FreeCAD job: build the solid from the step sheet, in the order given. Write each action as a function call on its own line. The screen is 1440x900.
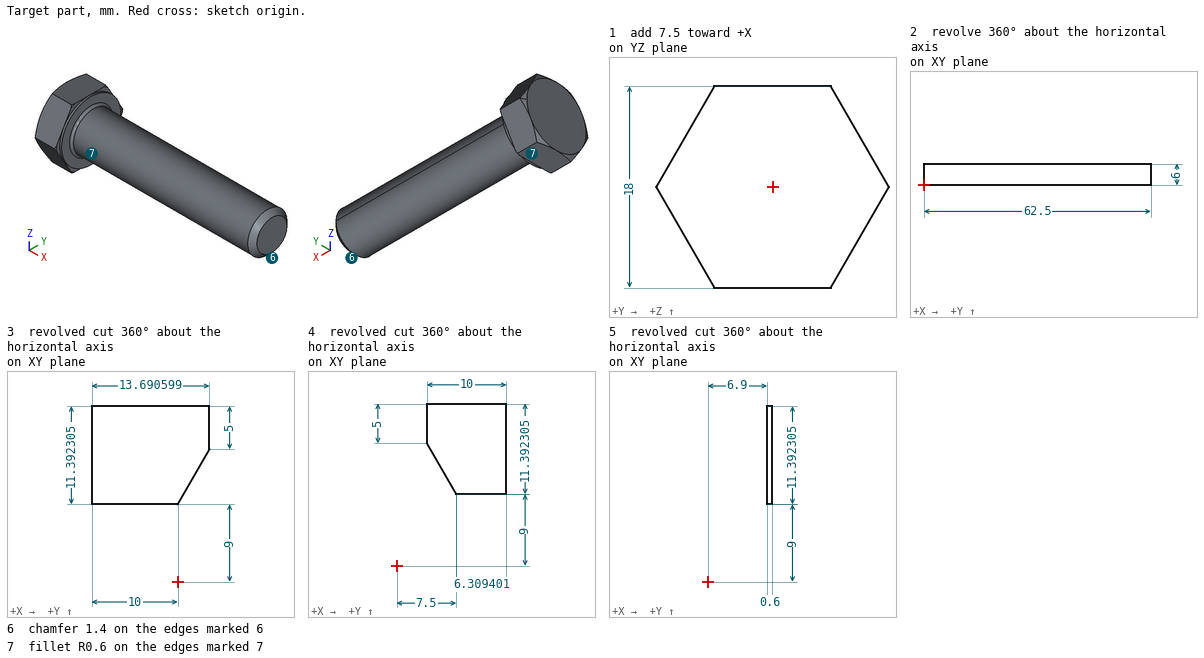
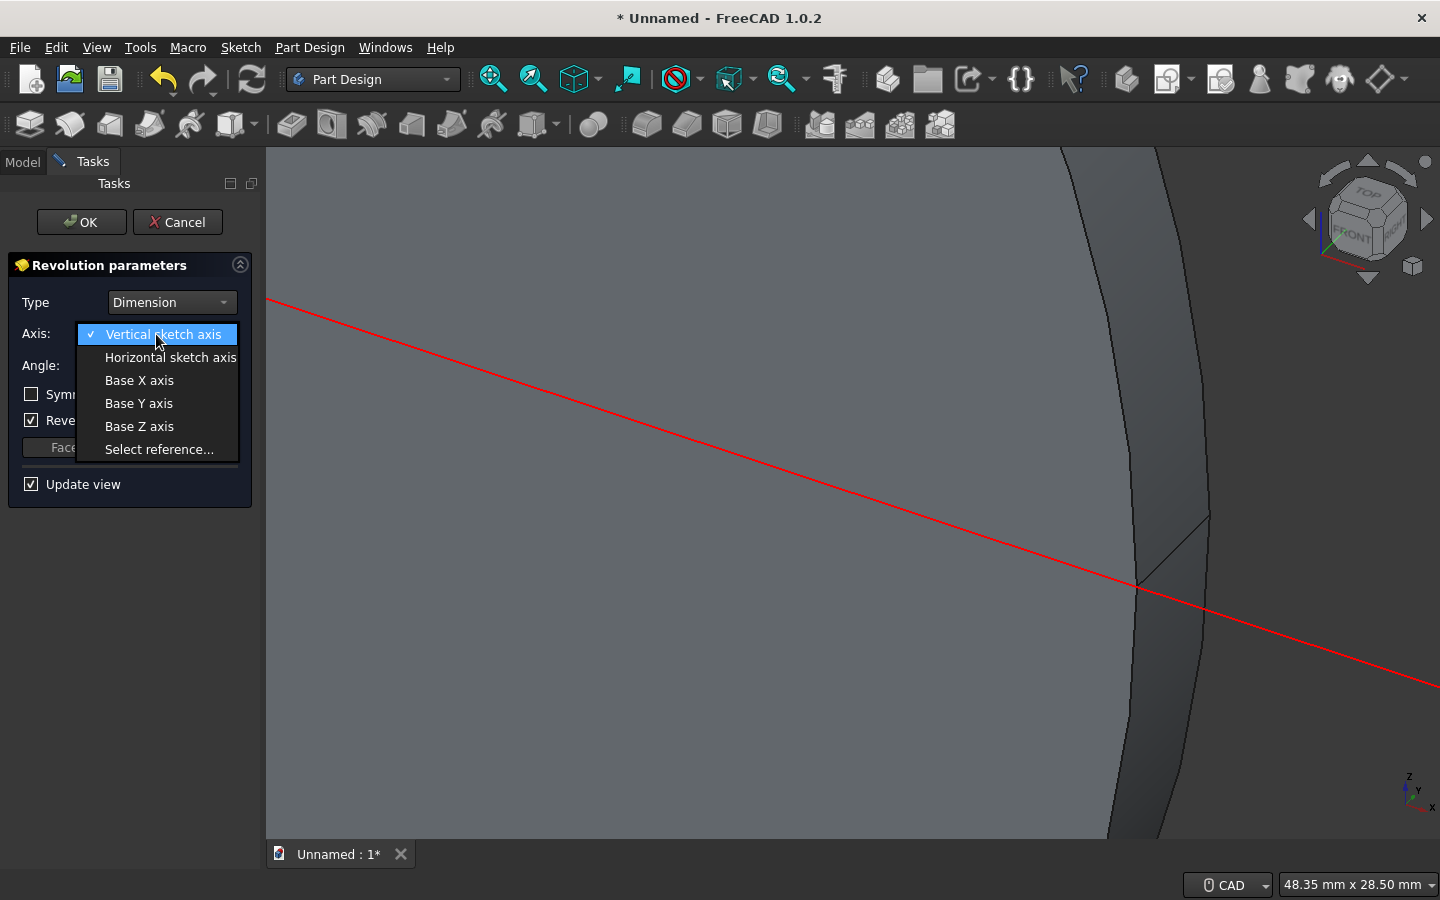
click(156, 358)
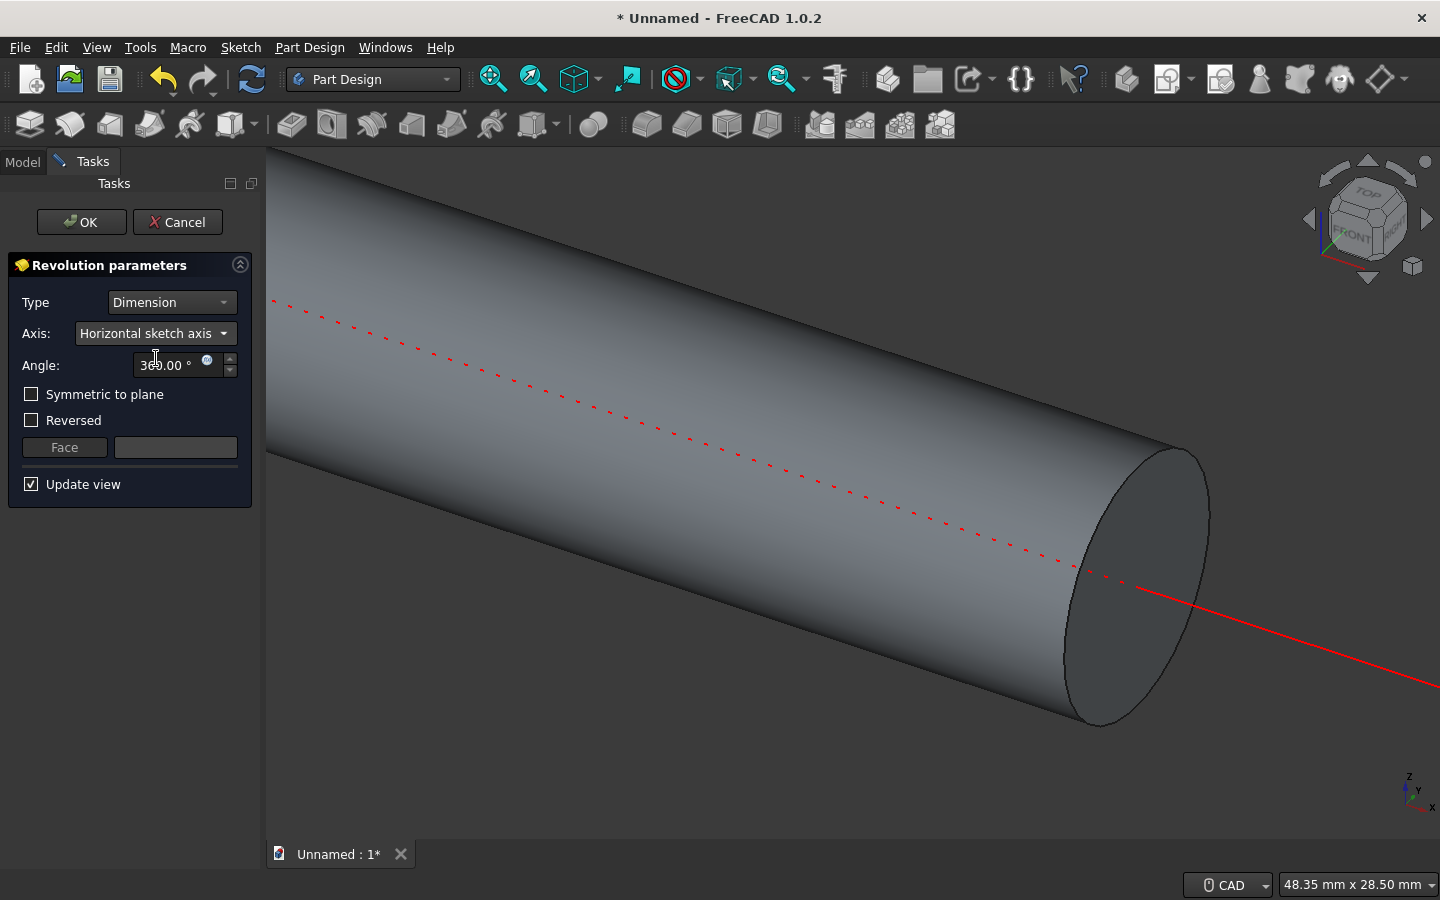
click(82, 222)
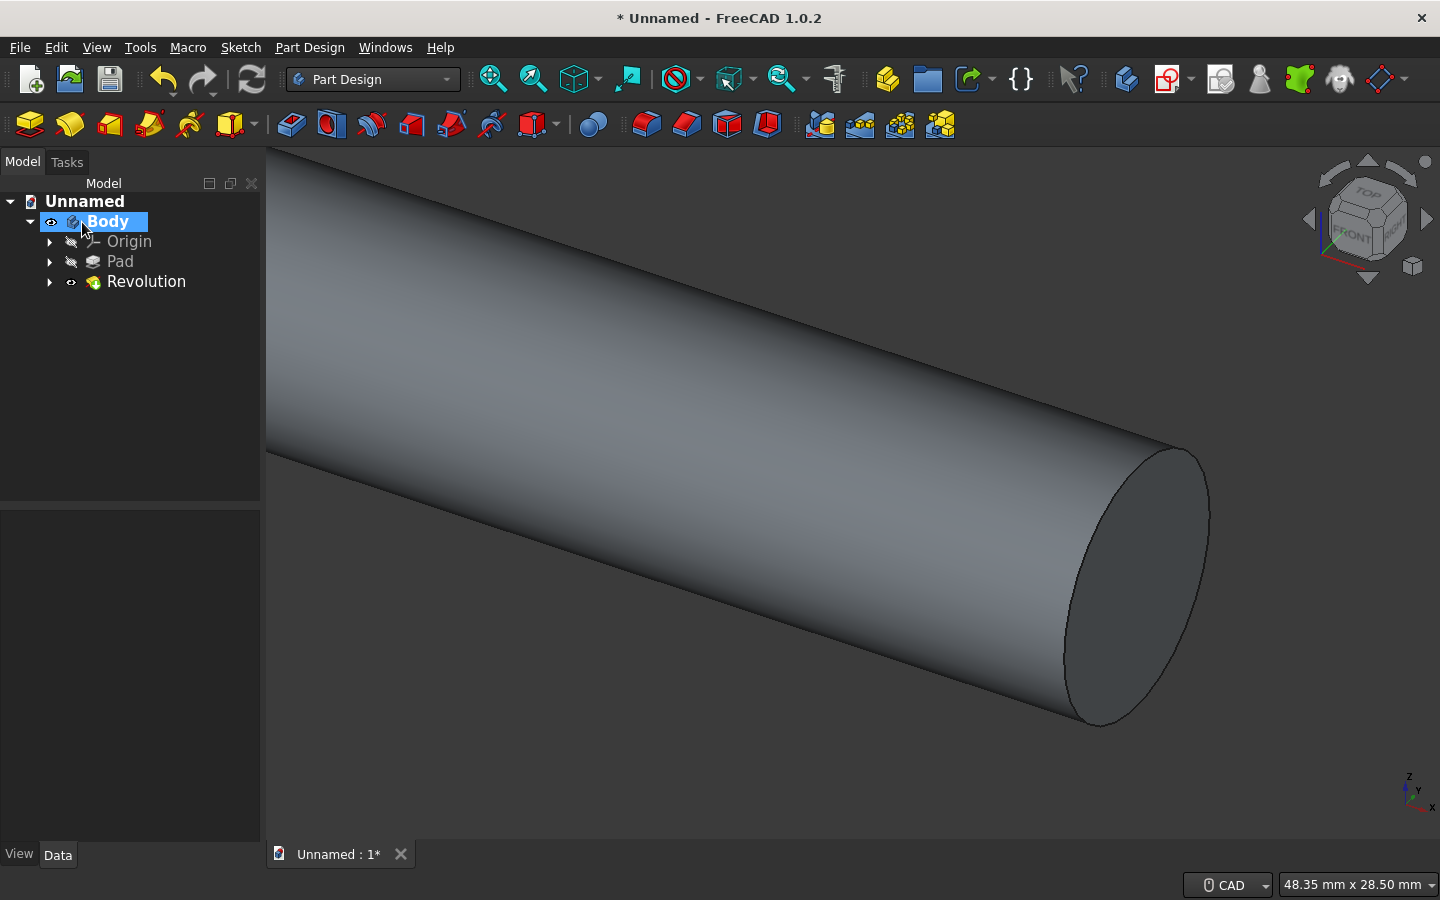
click(494, 80)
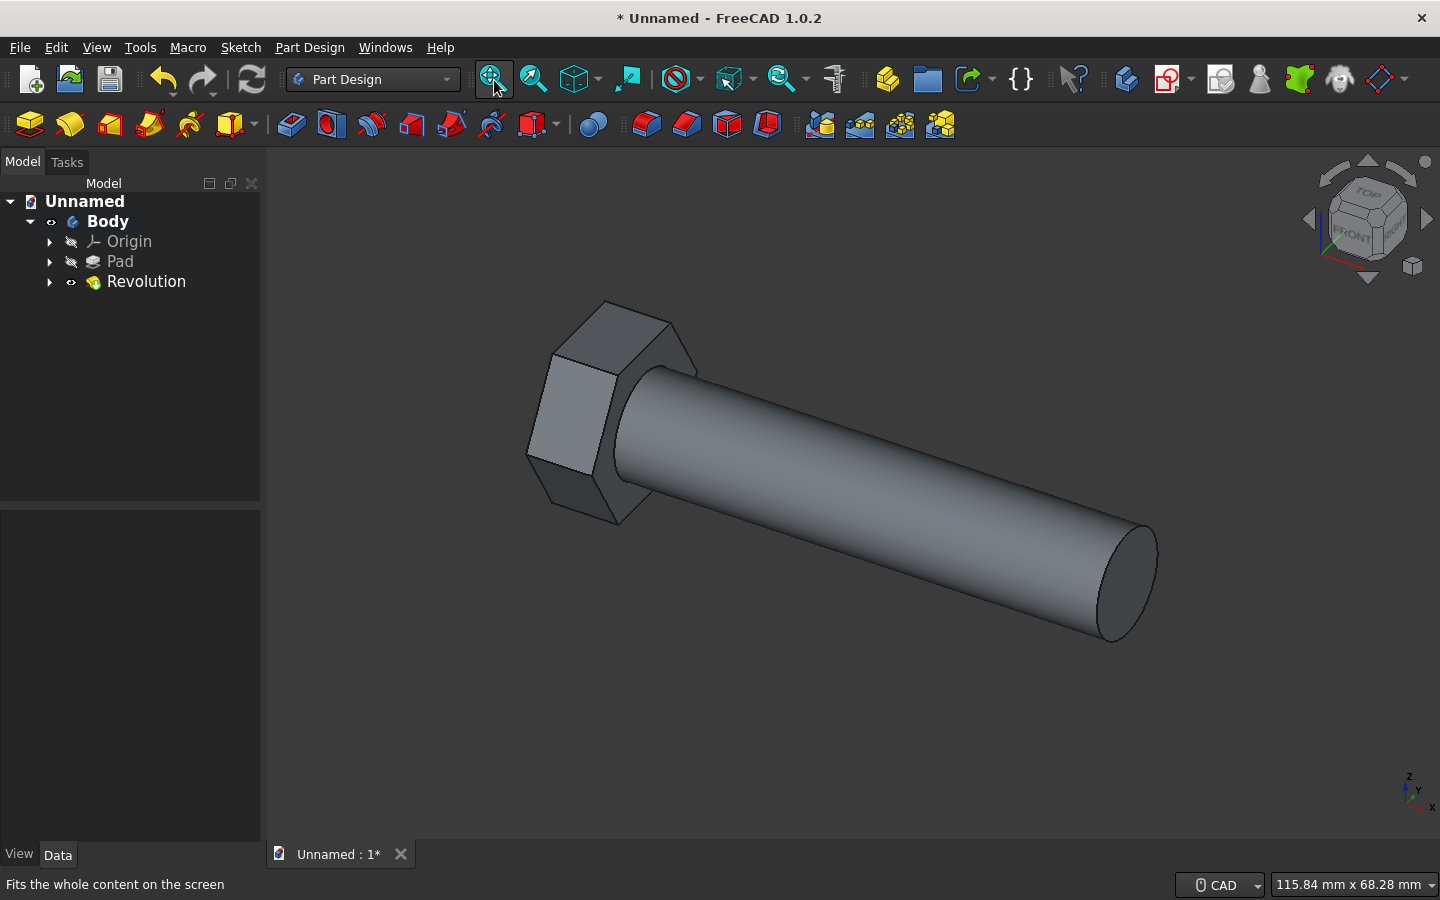
click(1168, 80)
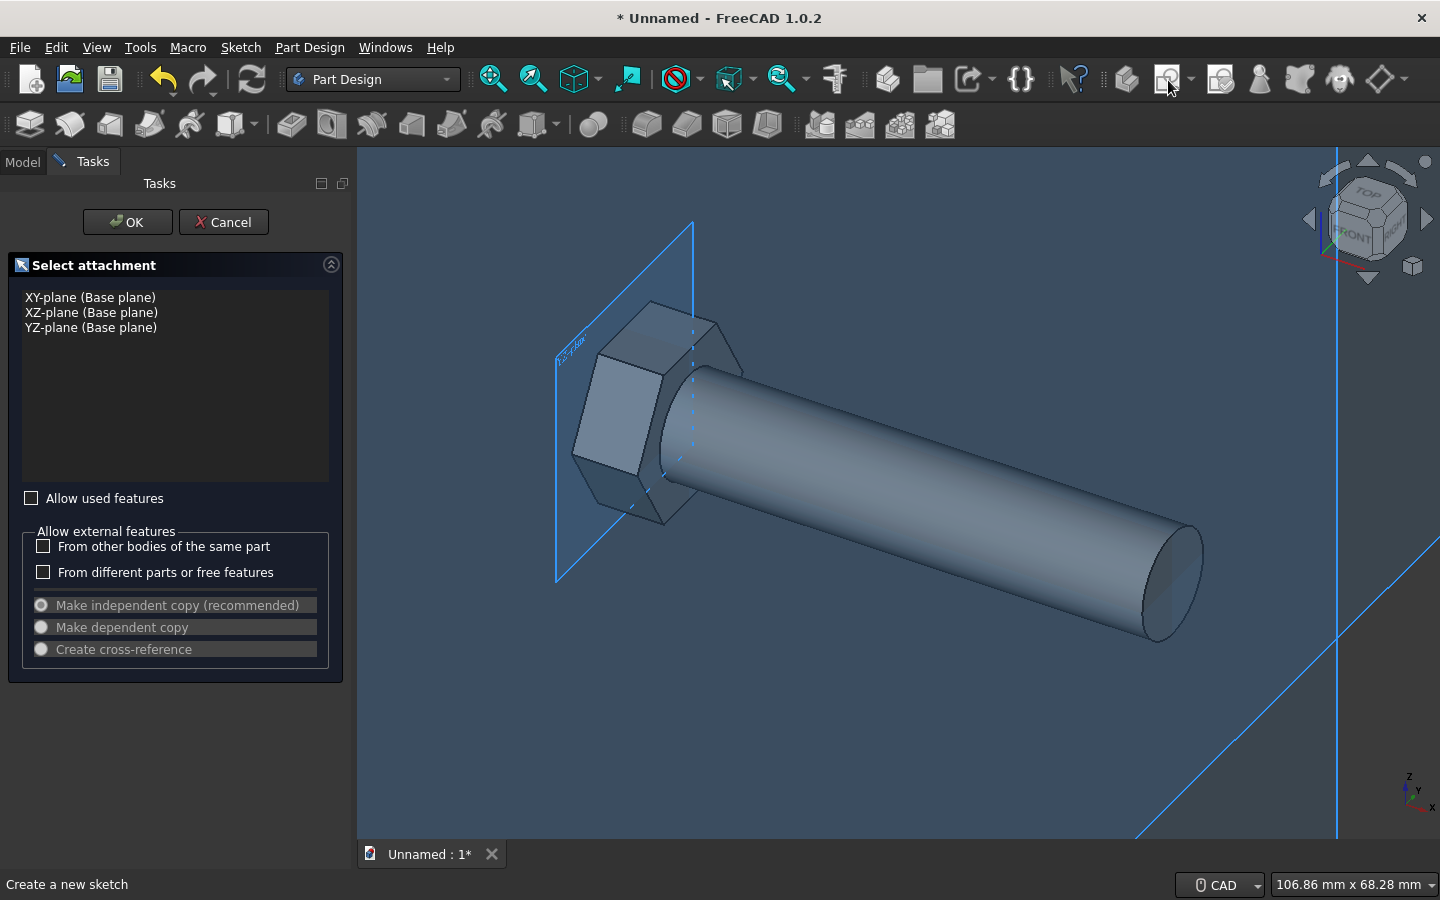
click(82, 298)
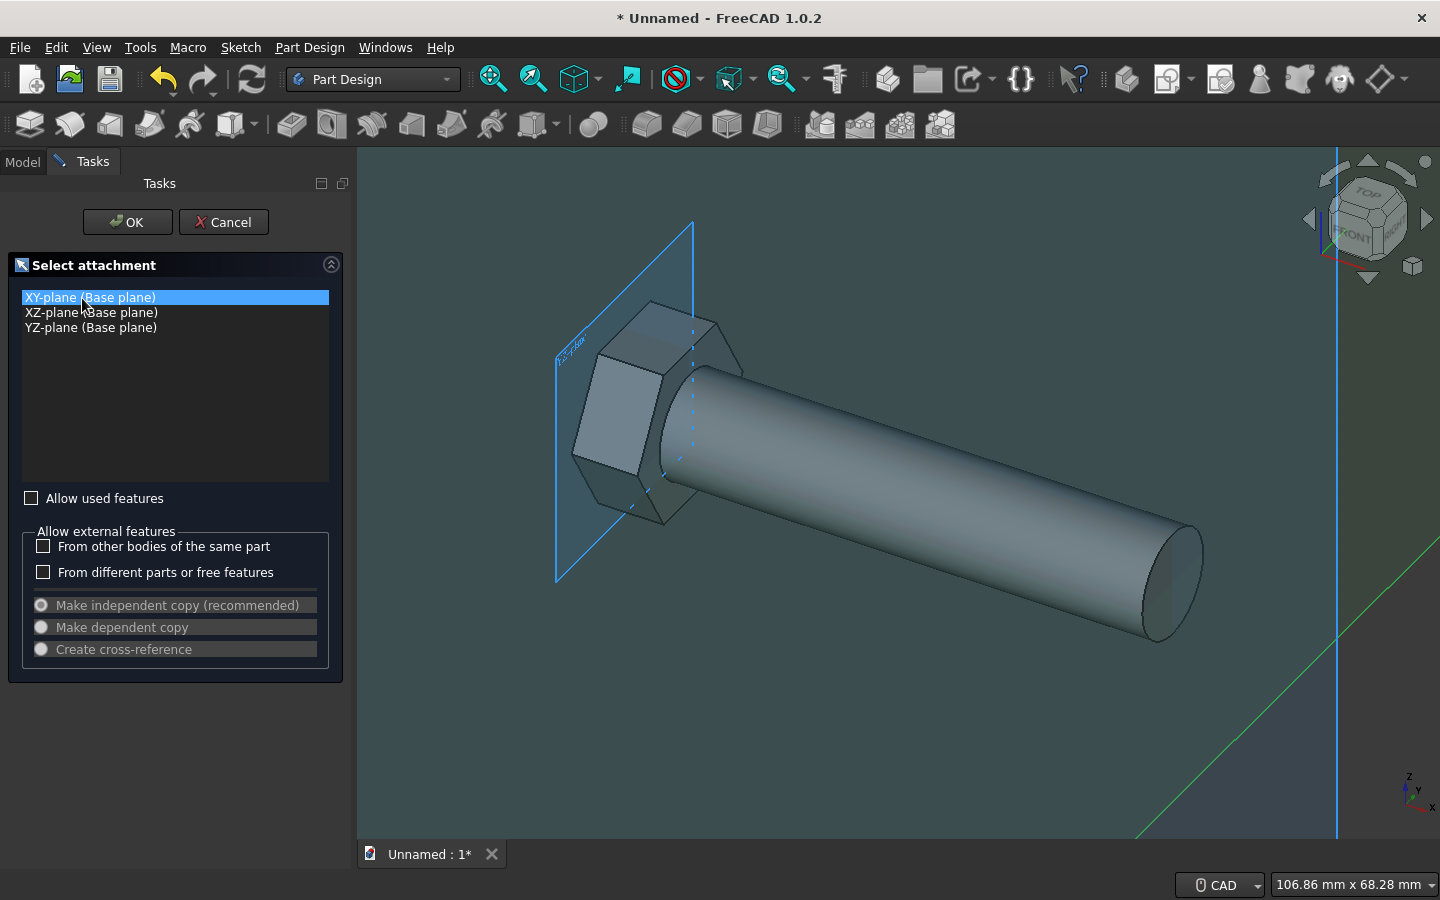
click(128, 222)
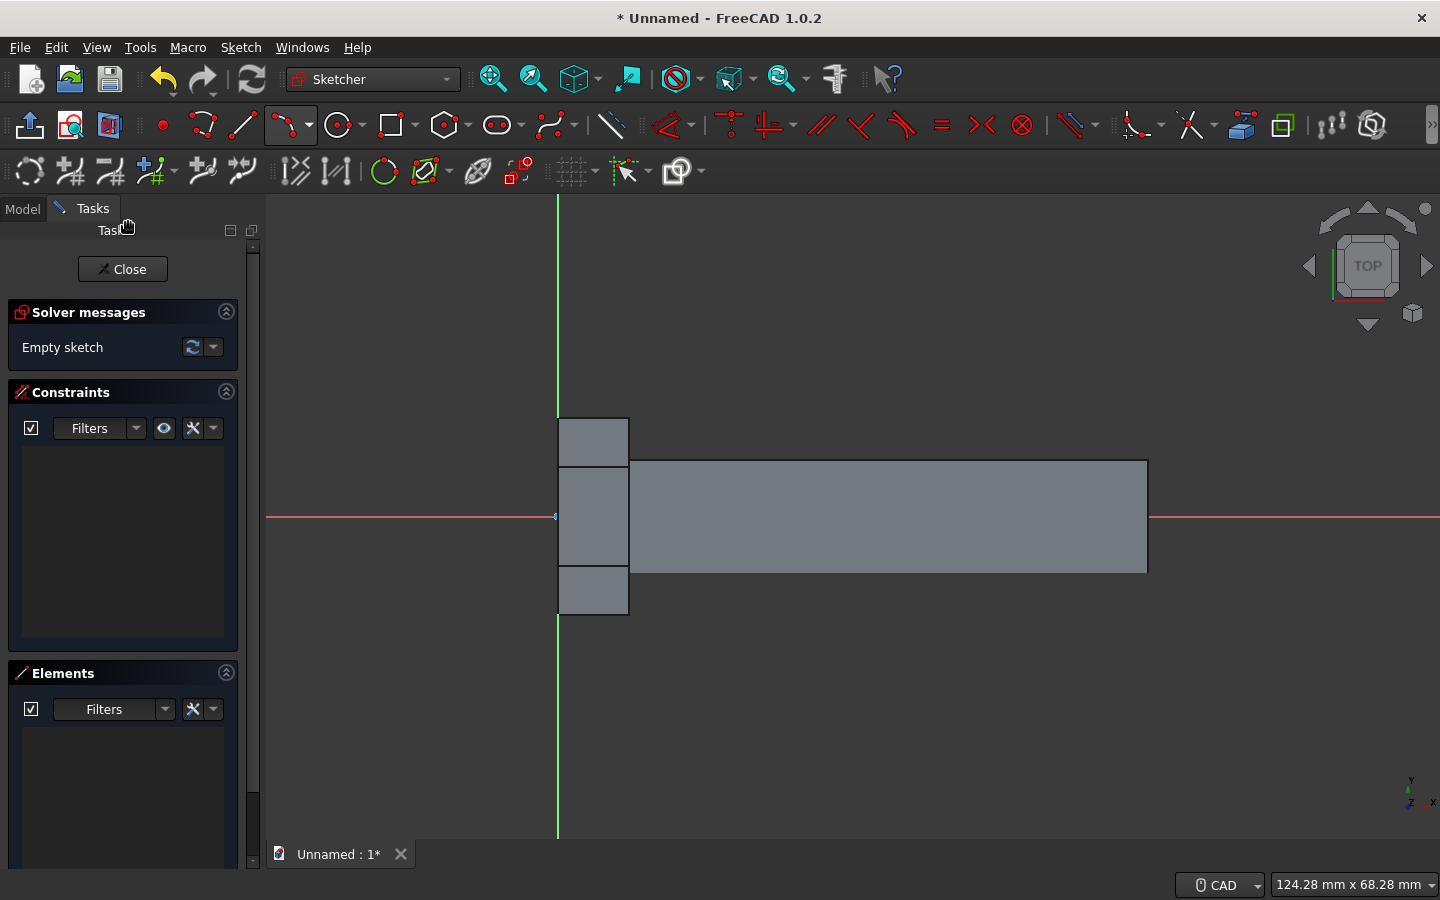
click(110, 126)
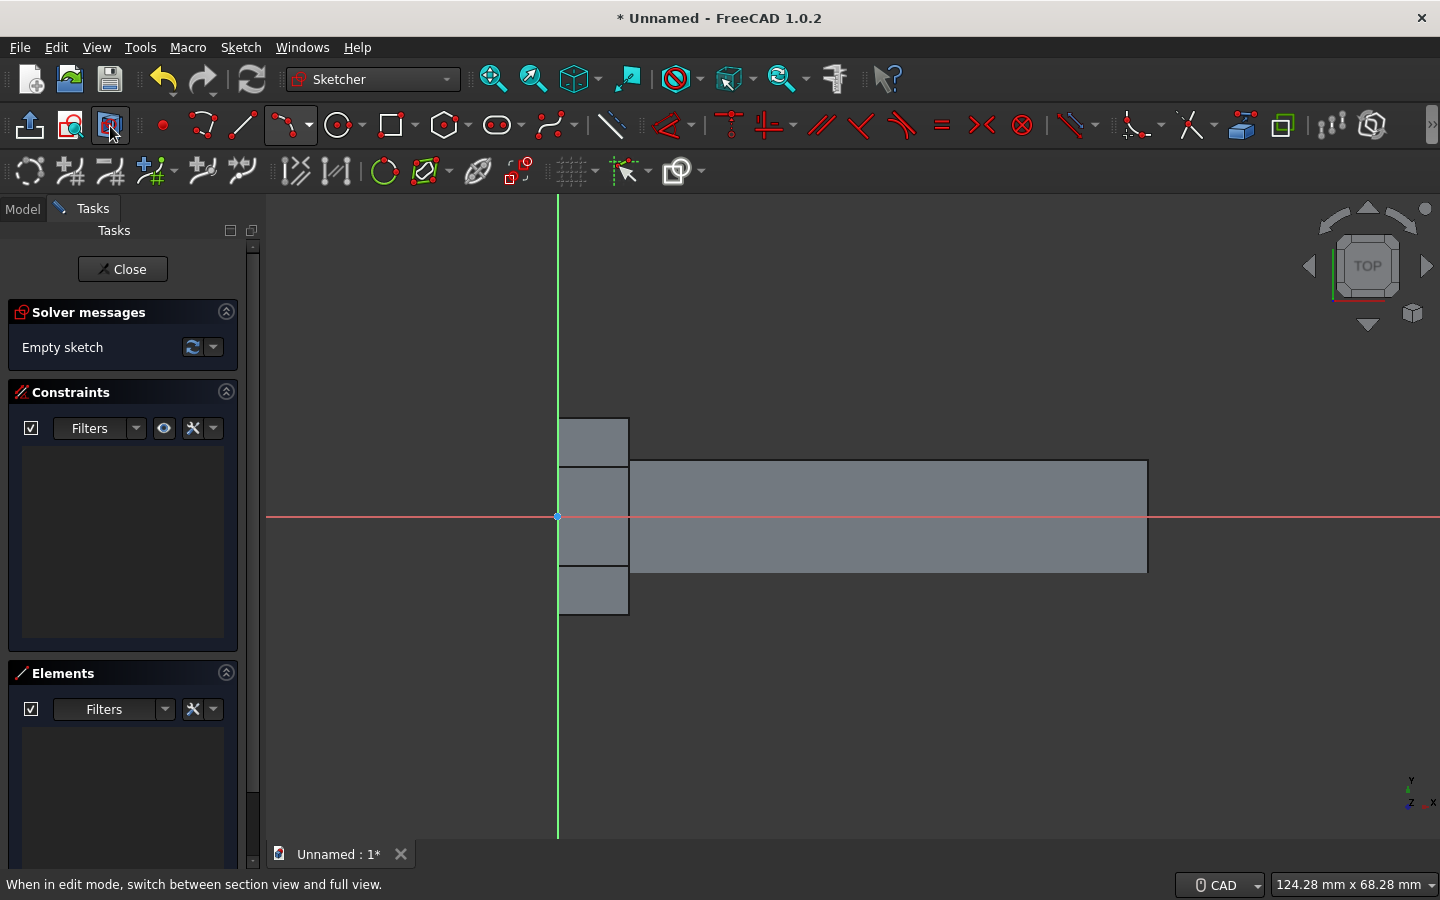
scroll(319, 342, up, 4)